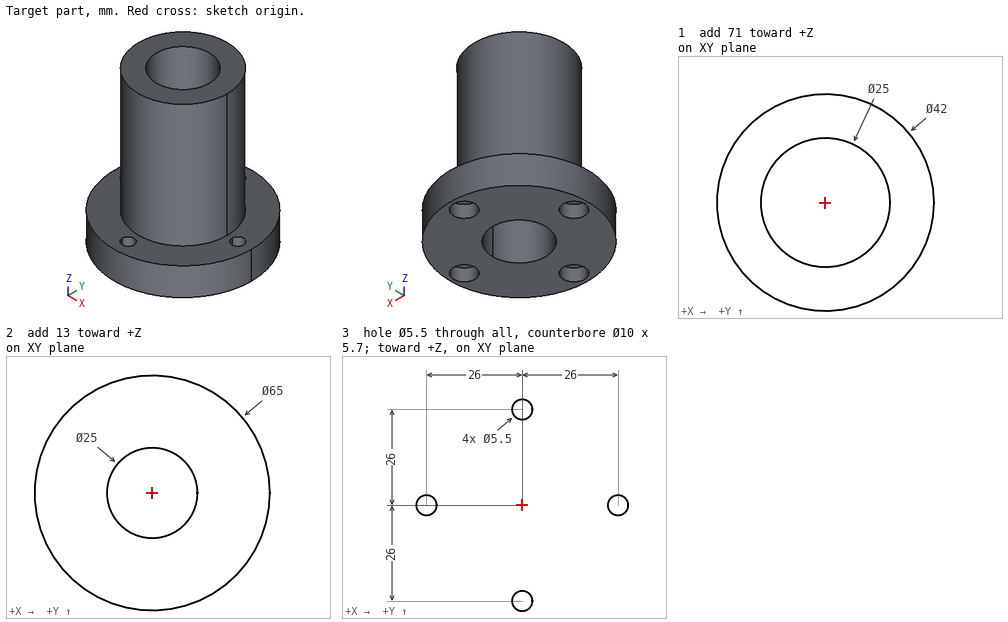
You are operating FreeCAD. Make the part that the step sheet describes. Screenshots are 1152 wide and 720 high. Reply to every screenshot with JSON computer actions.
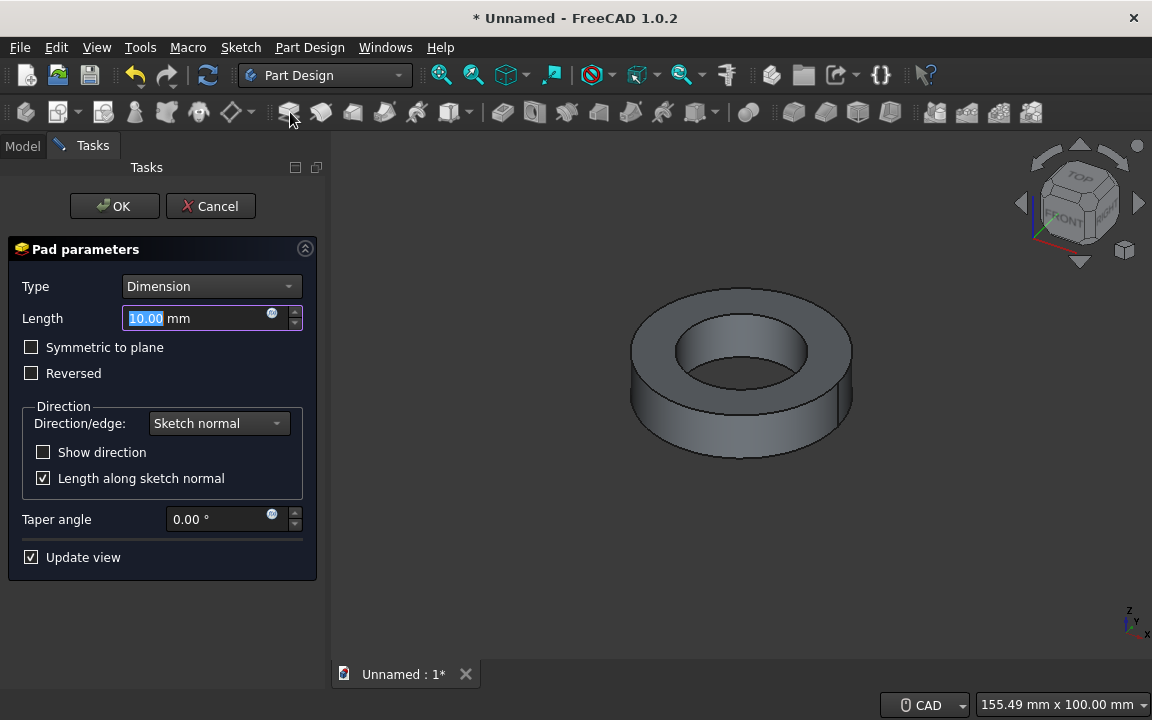
{"action": "type", "text": "71"}
{"action": "key", "text": "Tab"}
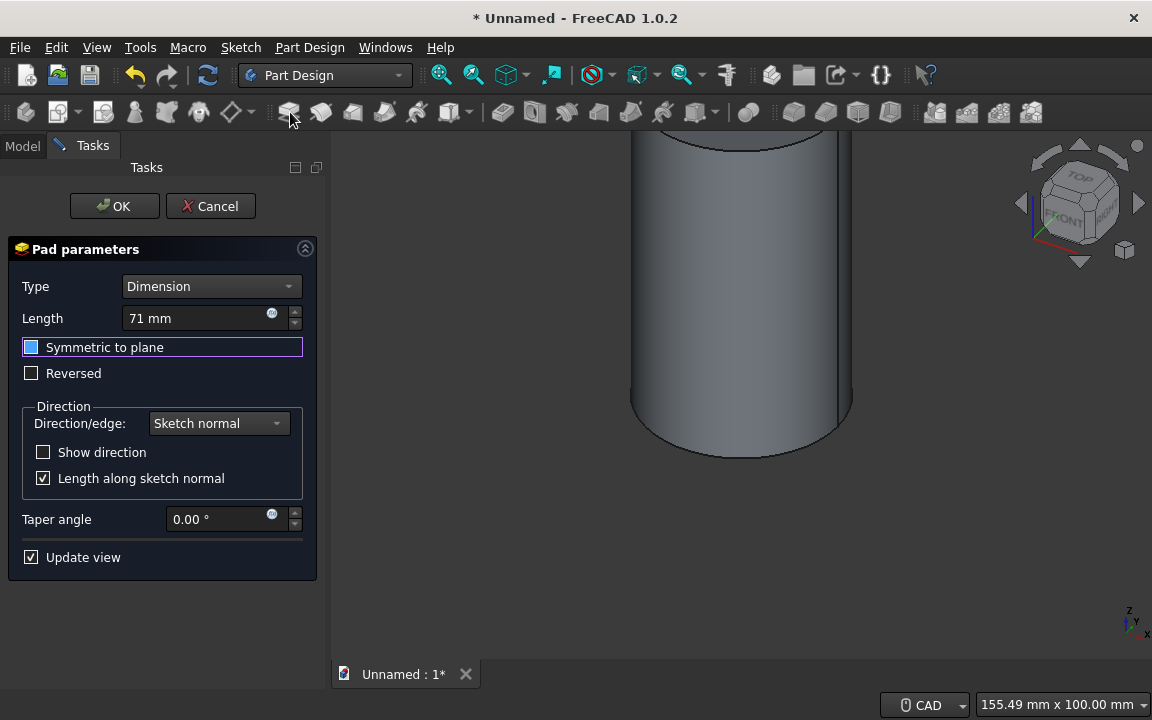
{"action": "left_click", "coordinate": [115, 206]}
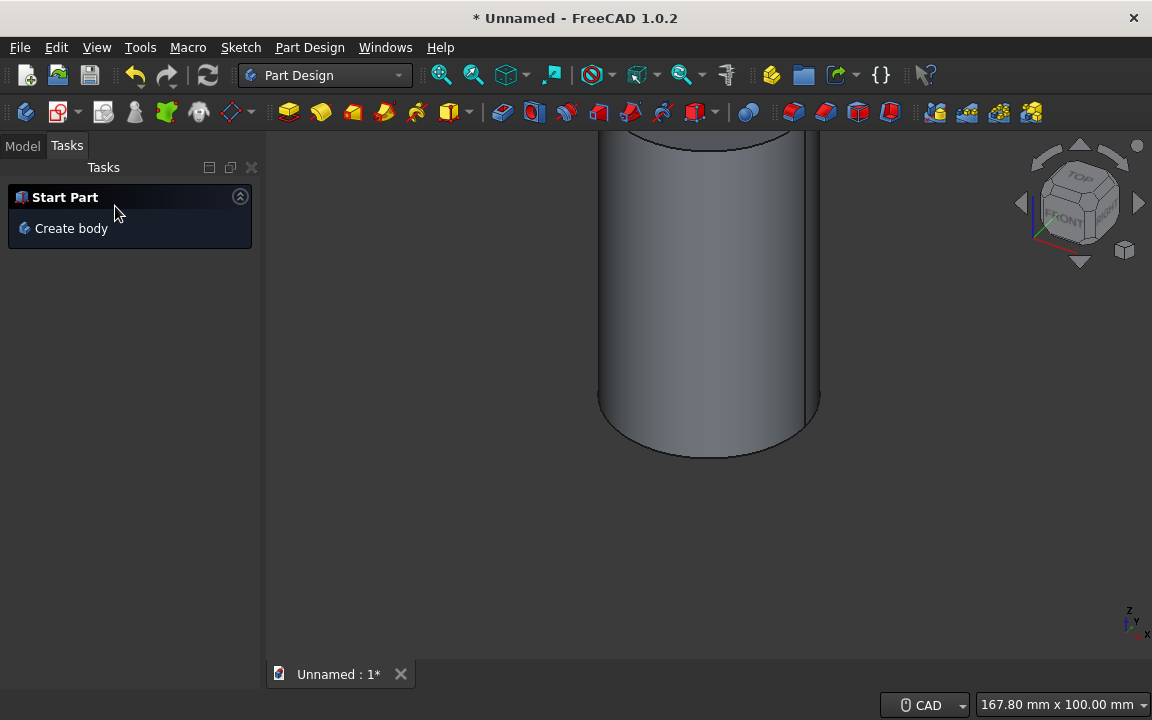
{"action": "left_click", "coordinate": [442, 76]}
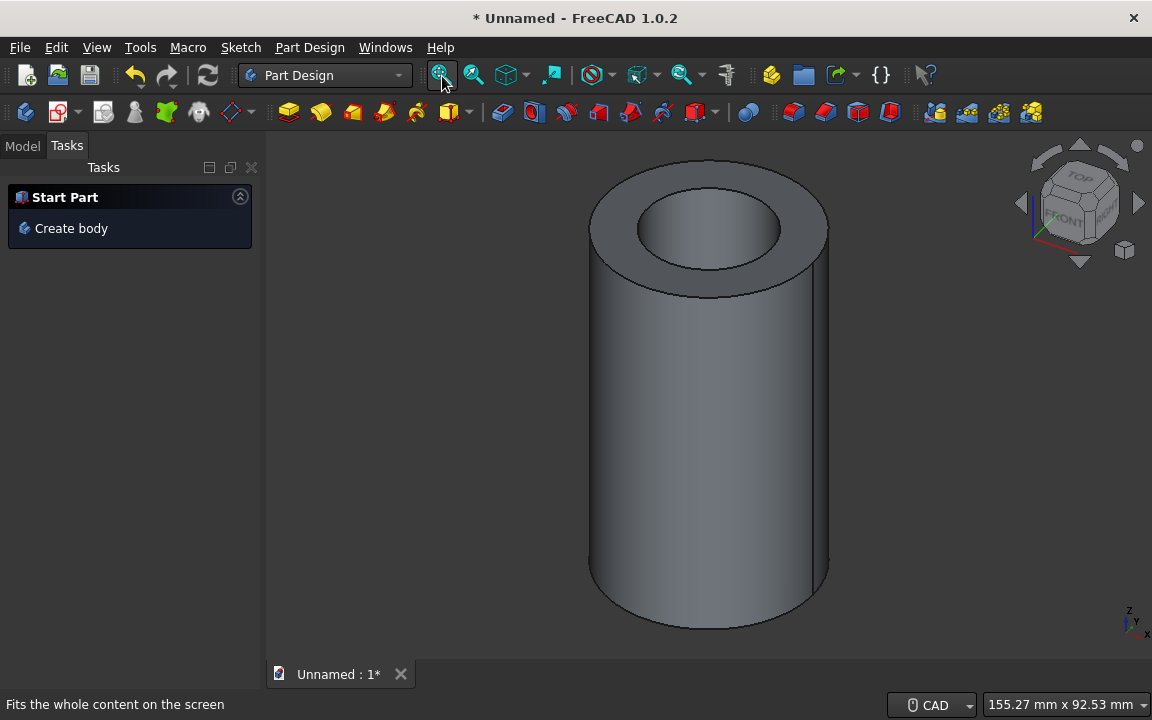
{"action": "left_click", "coordinate": [58, 112]}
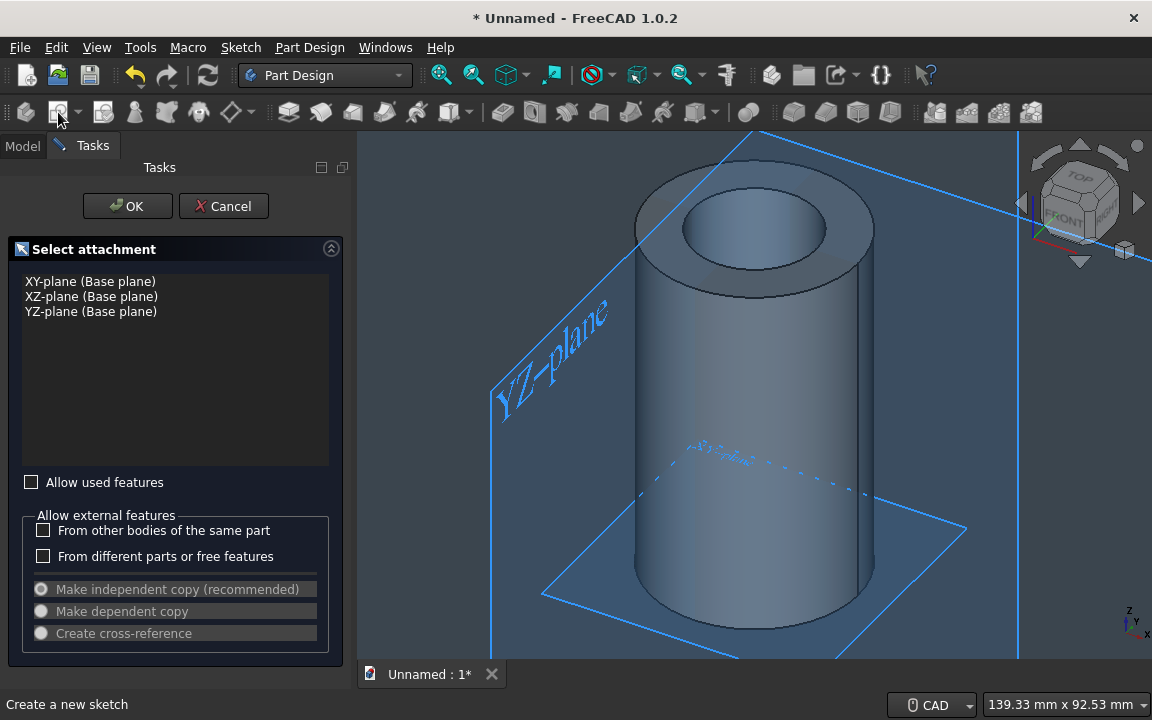
{"action": "left_click", "coordinate": [82, 282]}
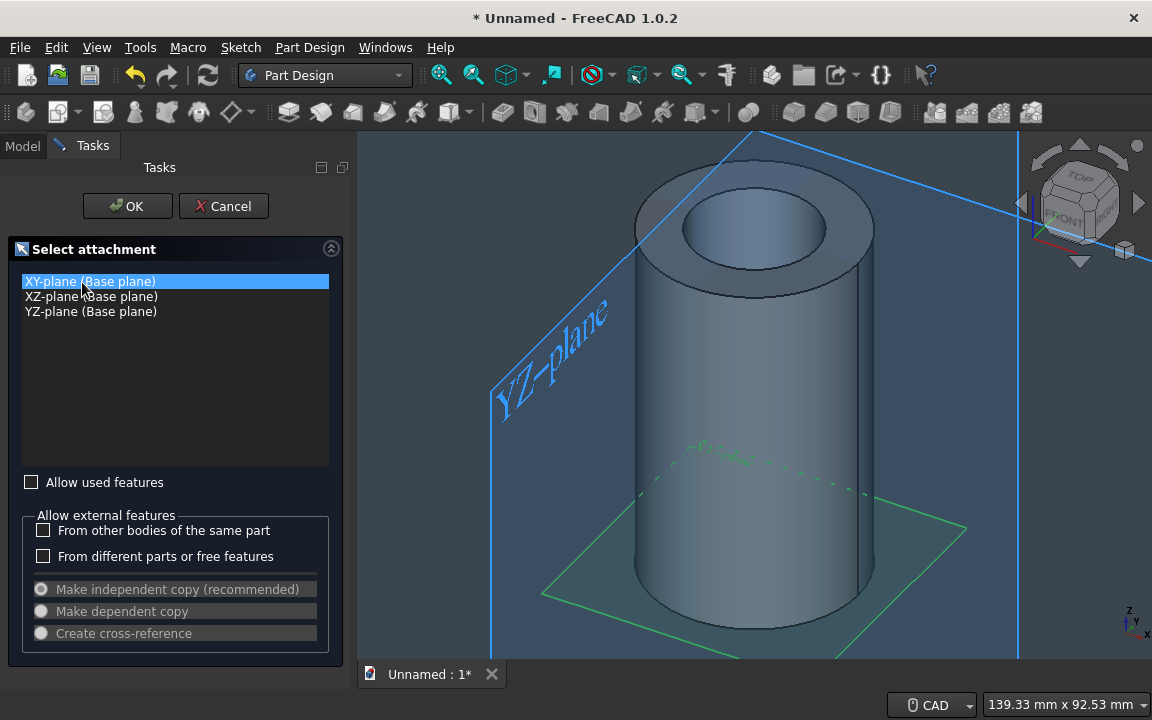
{"action": "left_click", "coordinate": [128, 206]}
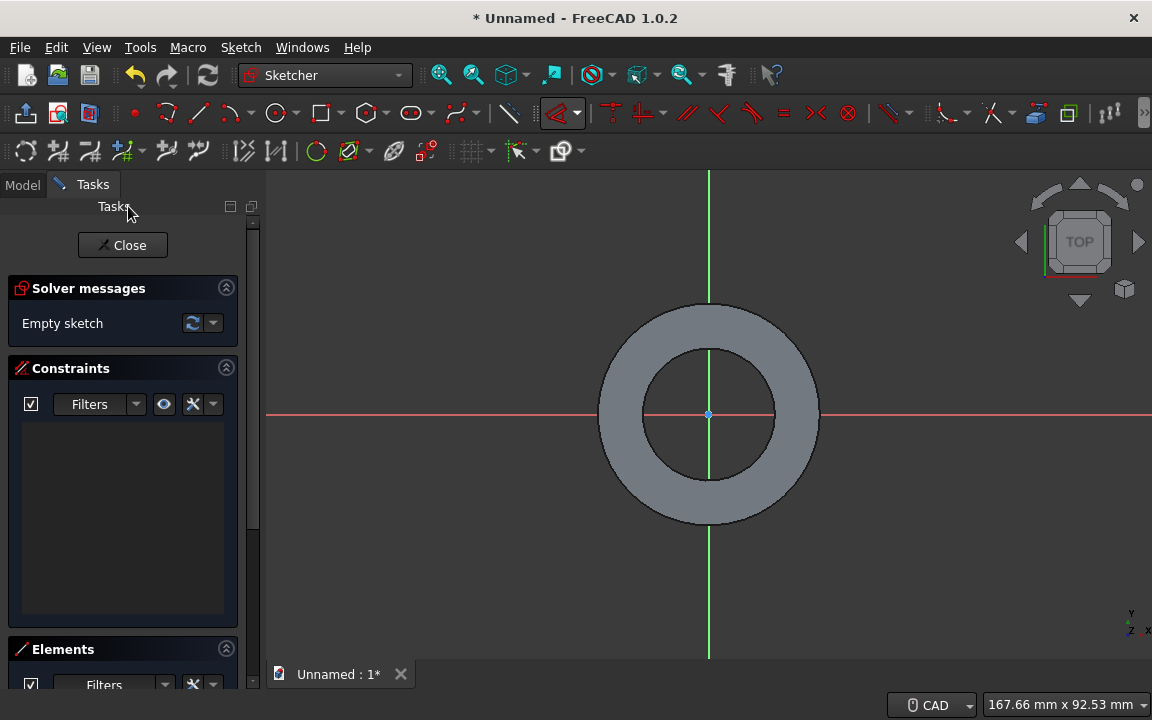
{"action": "left_click", "coordinate": [90, 114]}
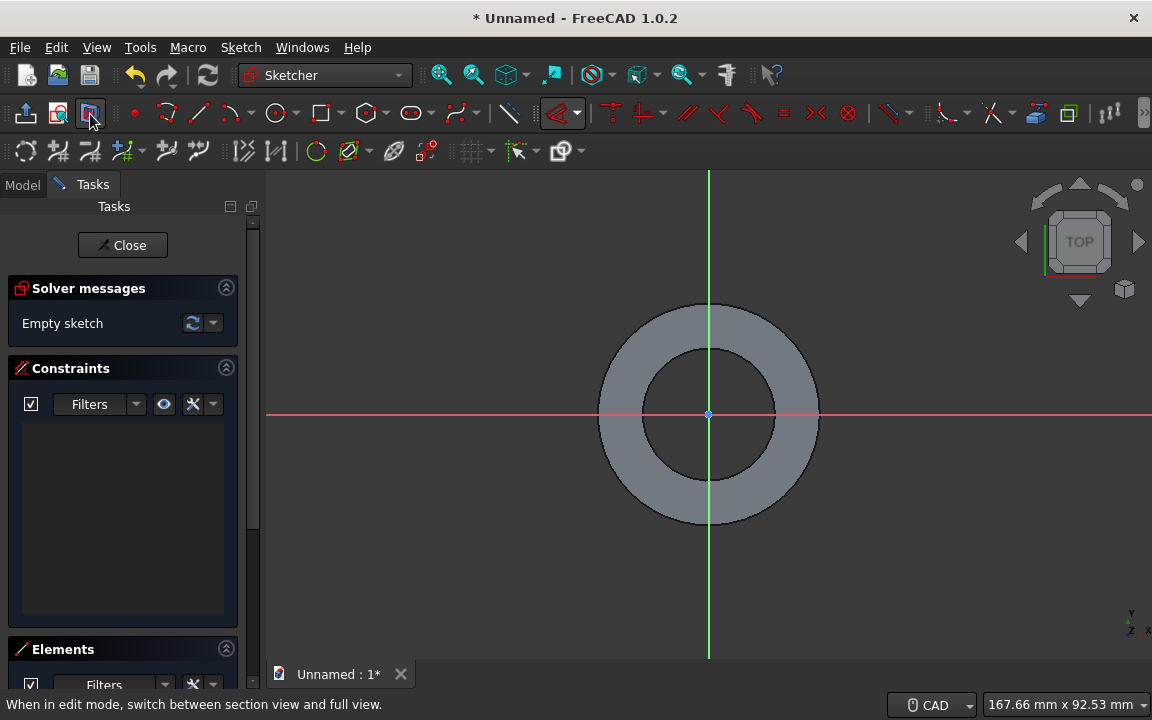
{"action": "left_click", "coordinate": [276, 114]}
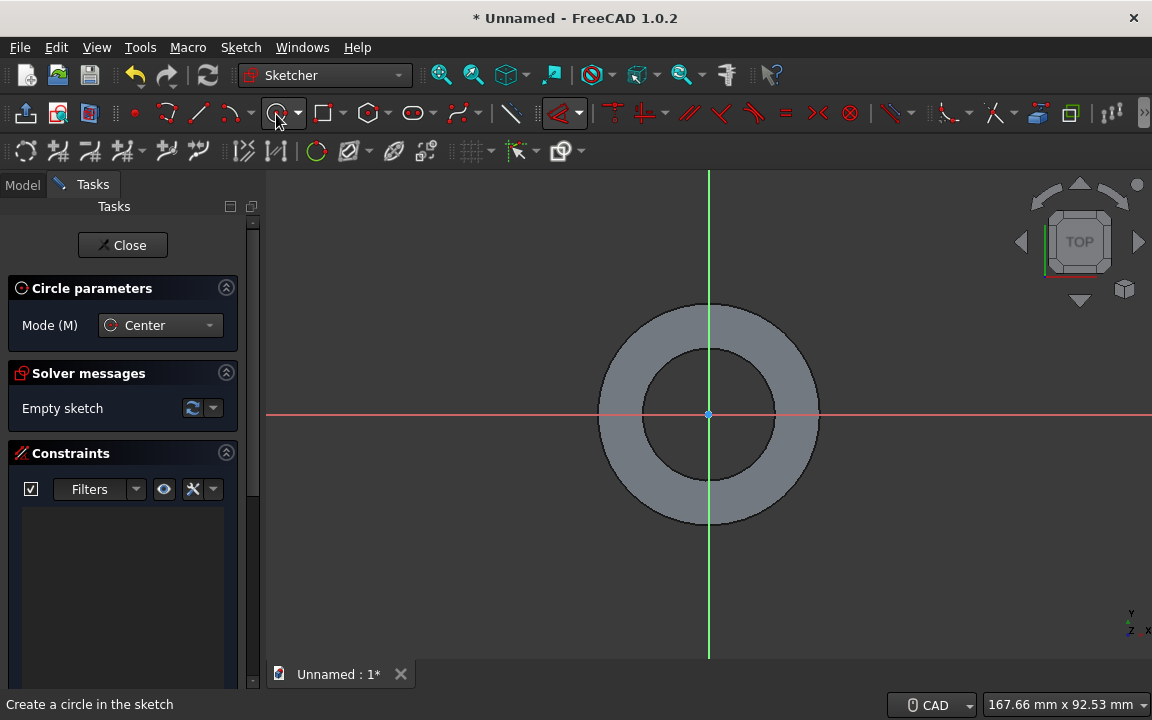
{"action": "left_click", "coordinate": [709, 414]}
{"action": "mouse_move", "coordinate": [830, 293]}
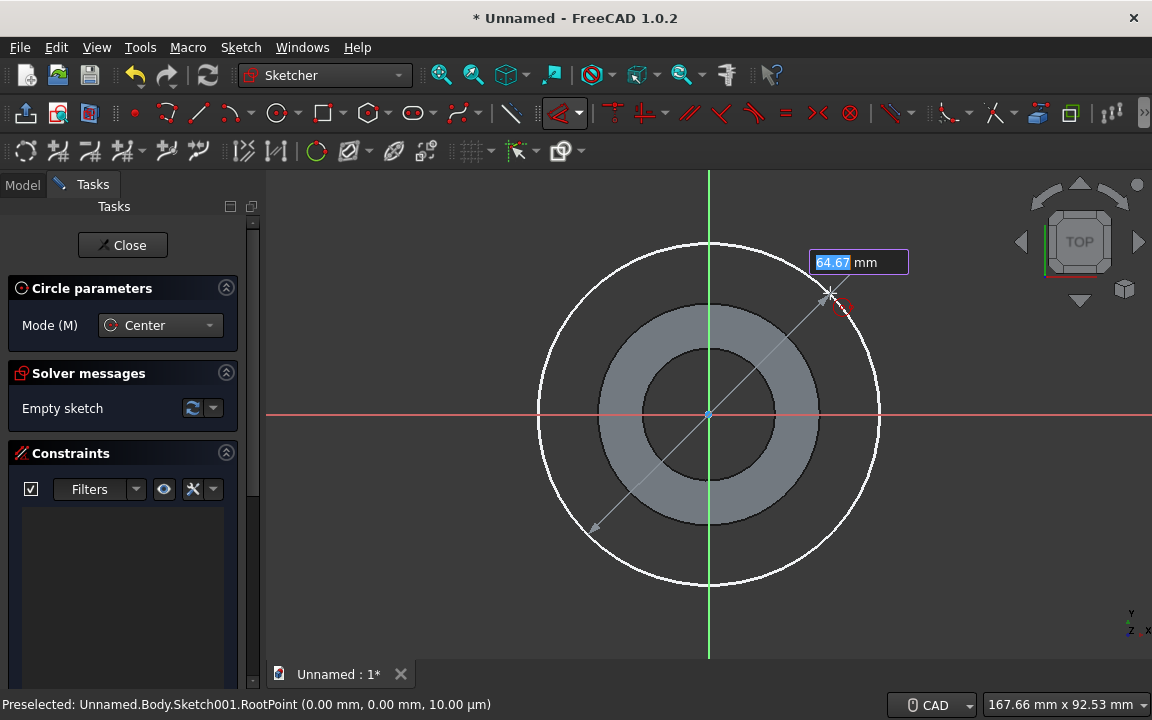
{"action": "type", "text": "65"}
{"action": "key", "text": "Return"}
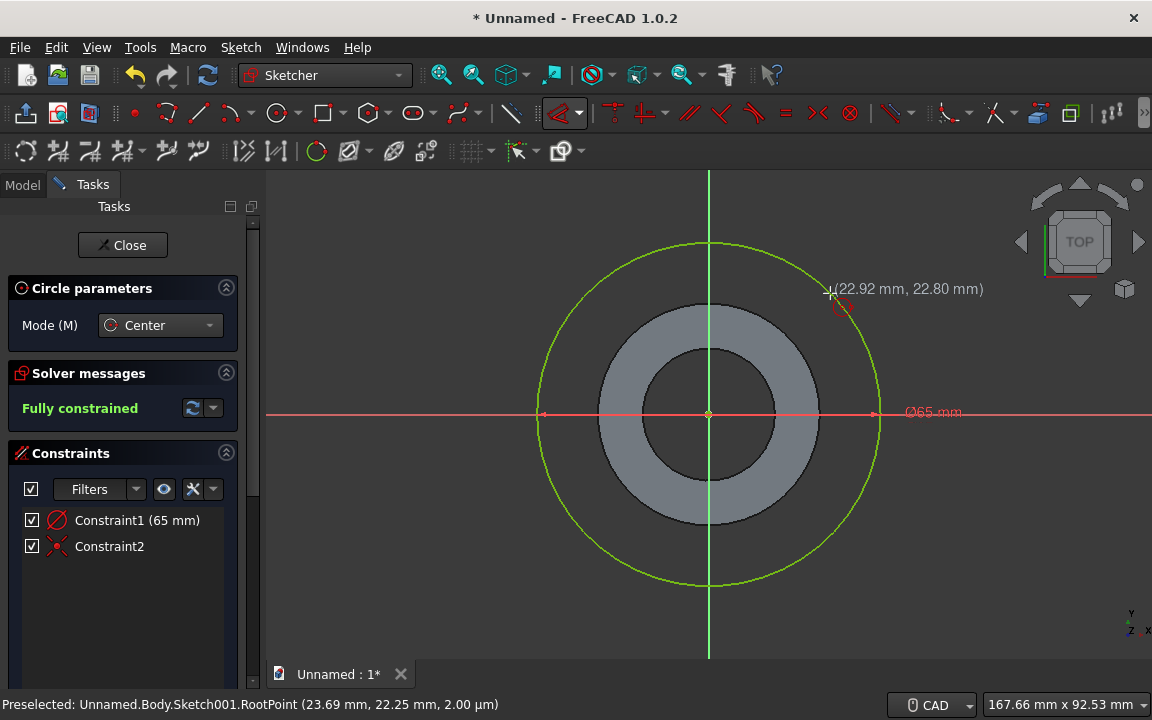
{"action": "left_click", "coordinate": [709, 414]}
{"action": "mouse_move", "coordinate": [756, 368]}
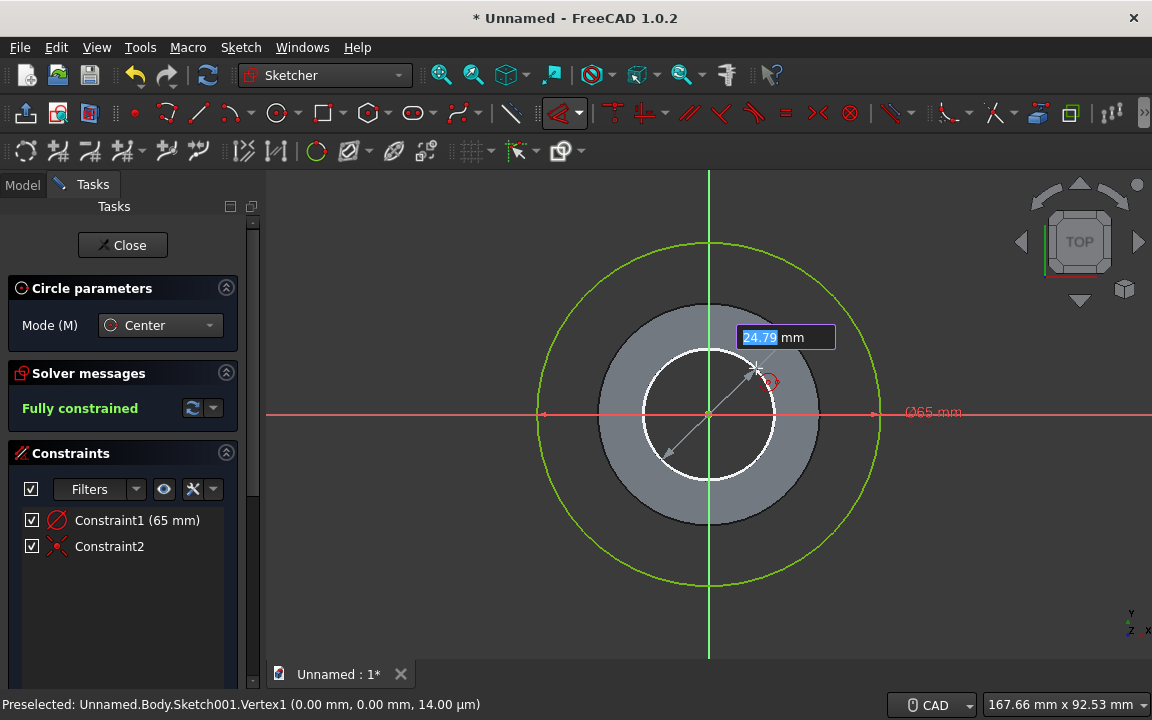
{"action": "type", "text": "25"}
{"action": "key", "text": "Return"}
{"action": "key", "text": "Escape"}